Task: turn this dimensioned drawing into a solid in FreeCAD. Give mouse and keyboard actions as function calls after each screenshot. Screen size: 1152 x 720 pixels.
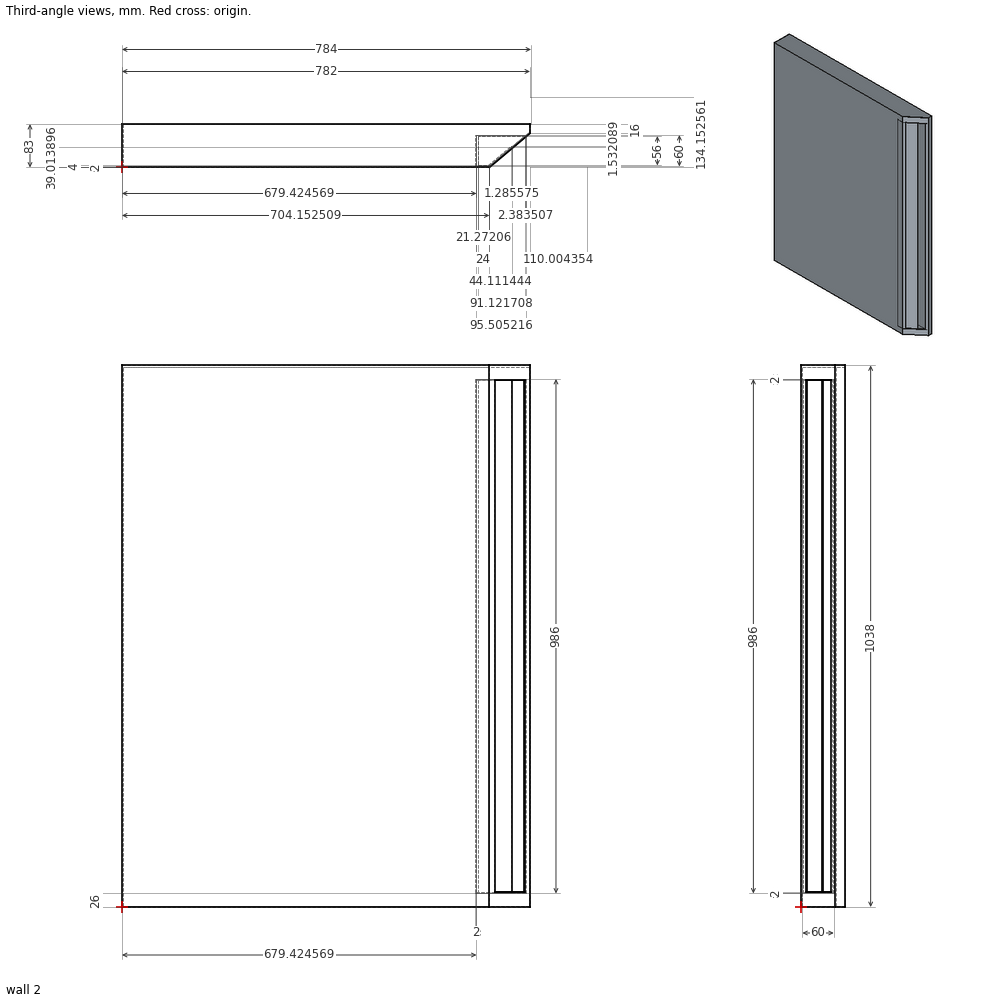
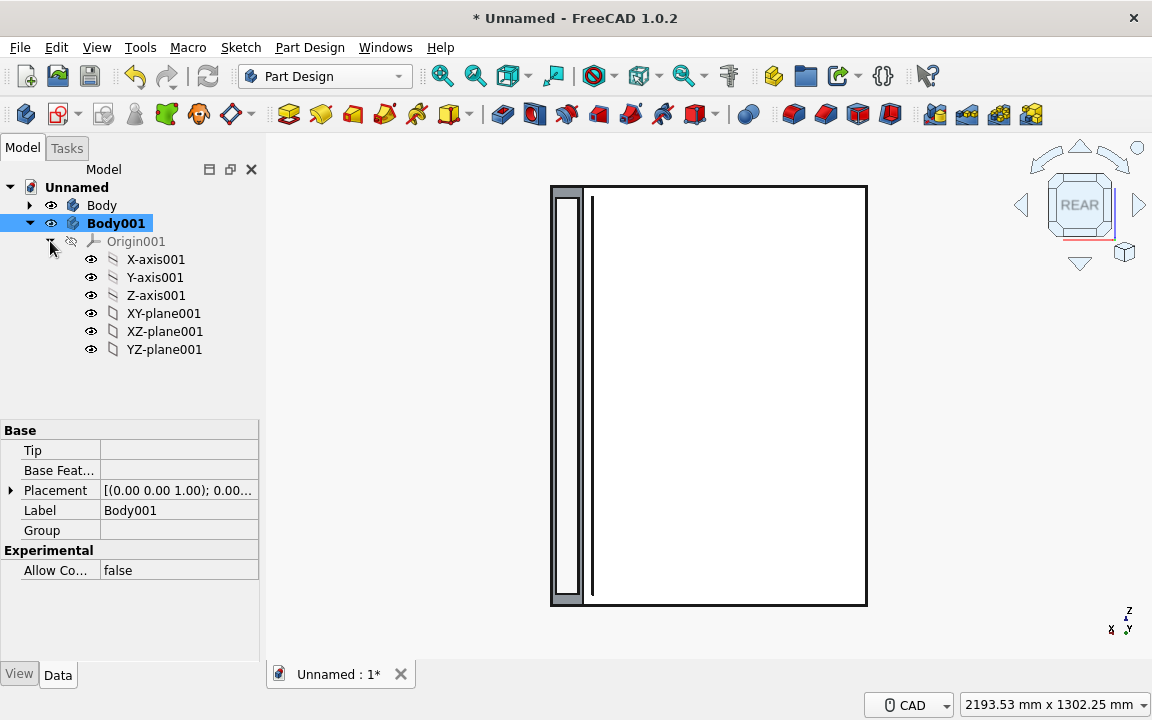
click(136, 313)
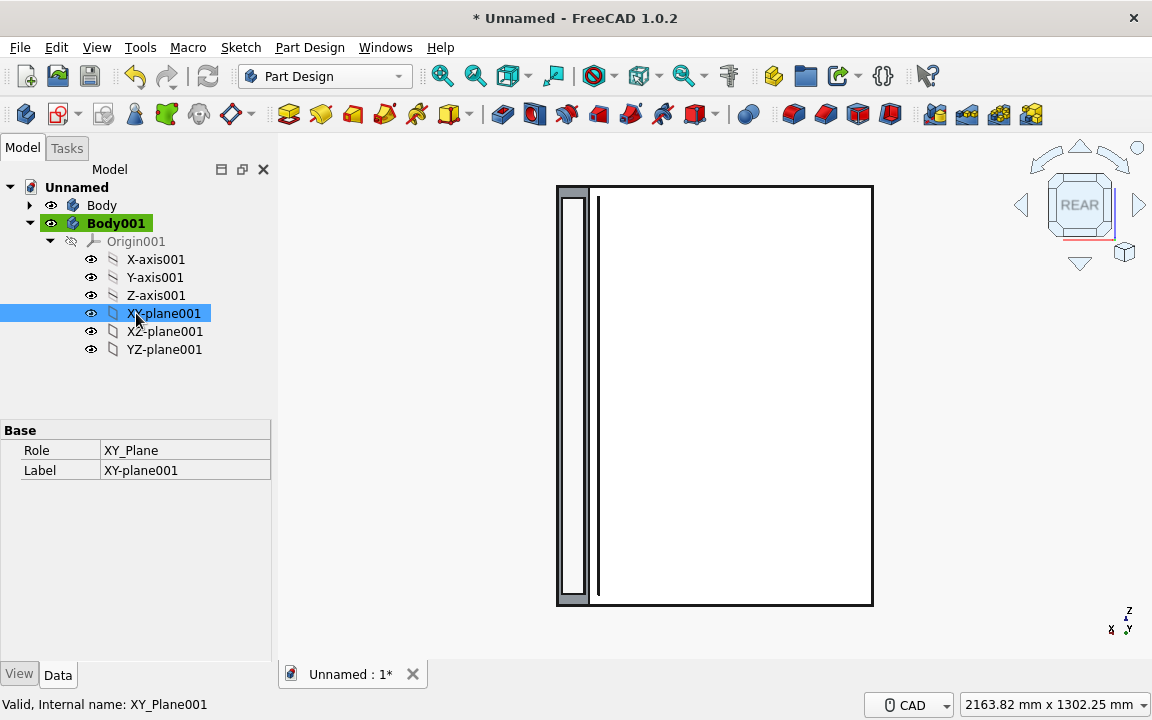
click(232, 114)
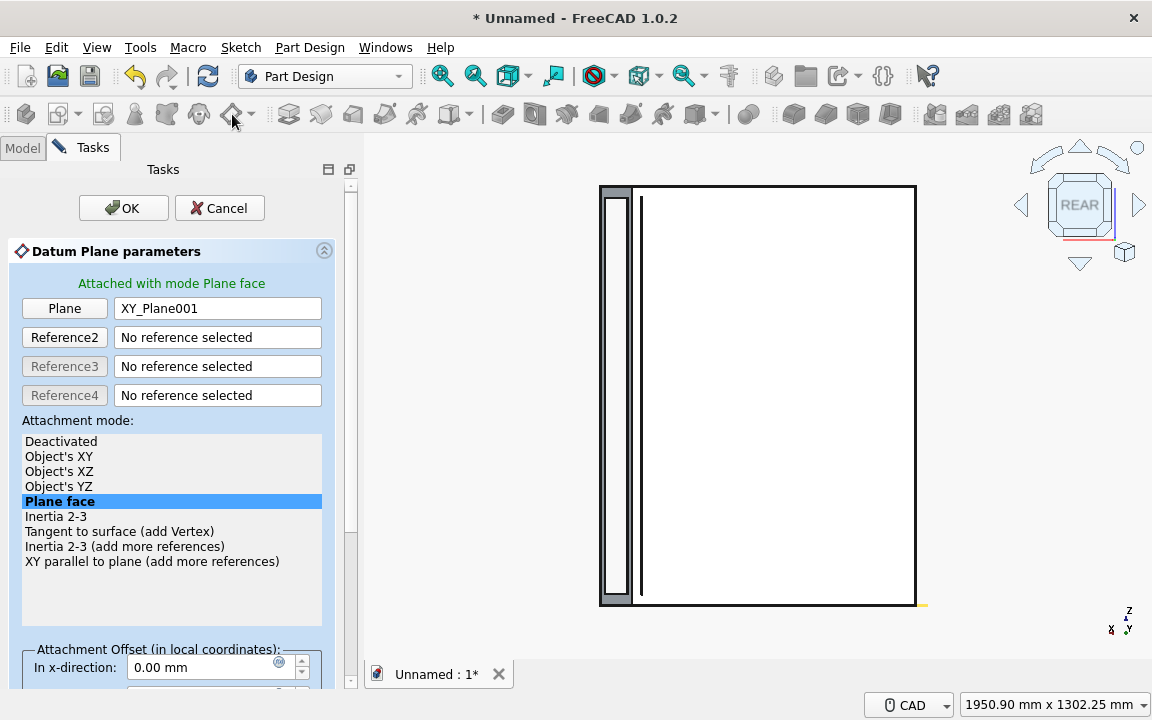
scroll(351, 434, down, 2)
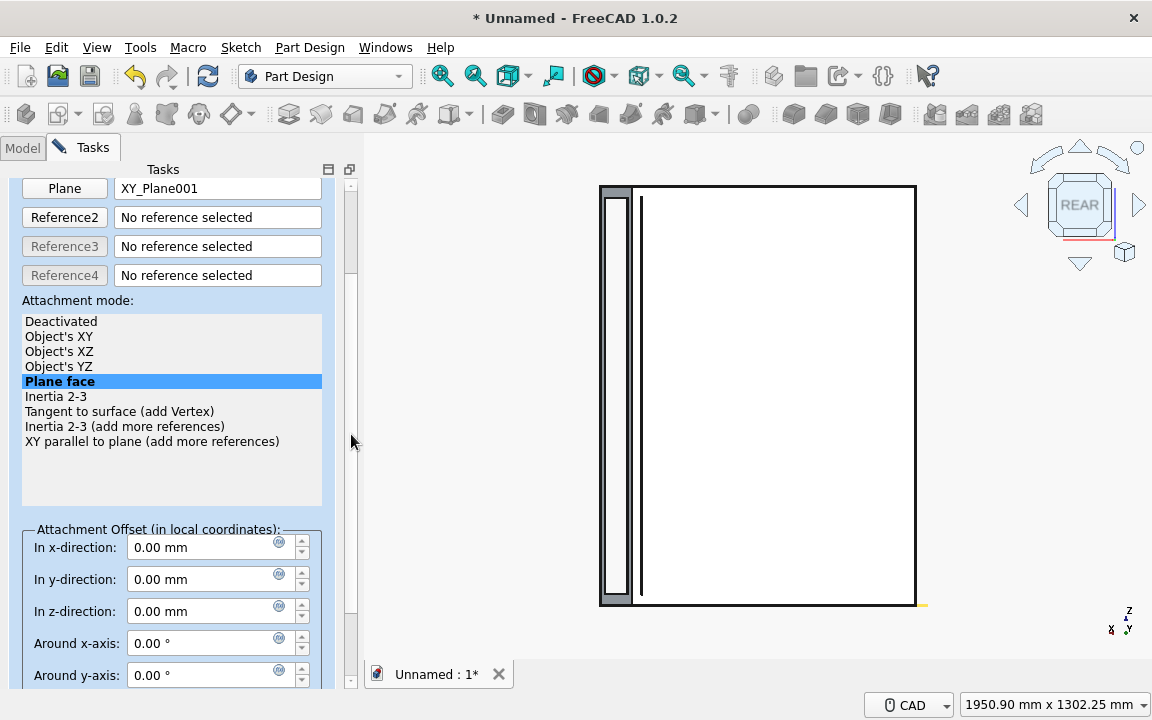
triple_click(210, 611)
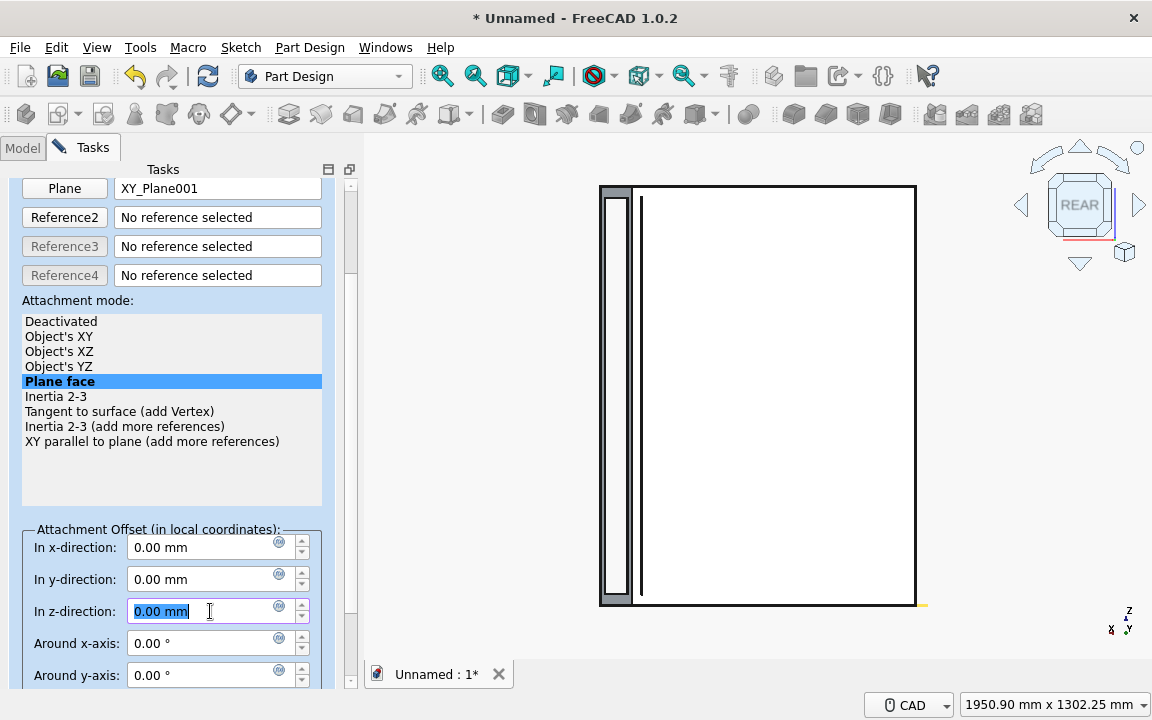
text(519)
key(Tab)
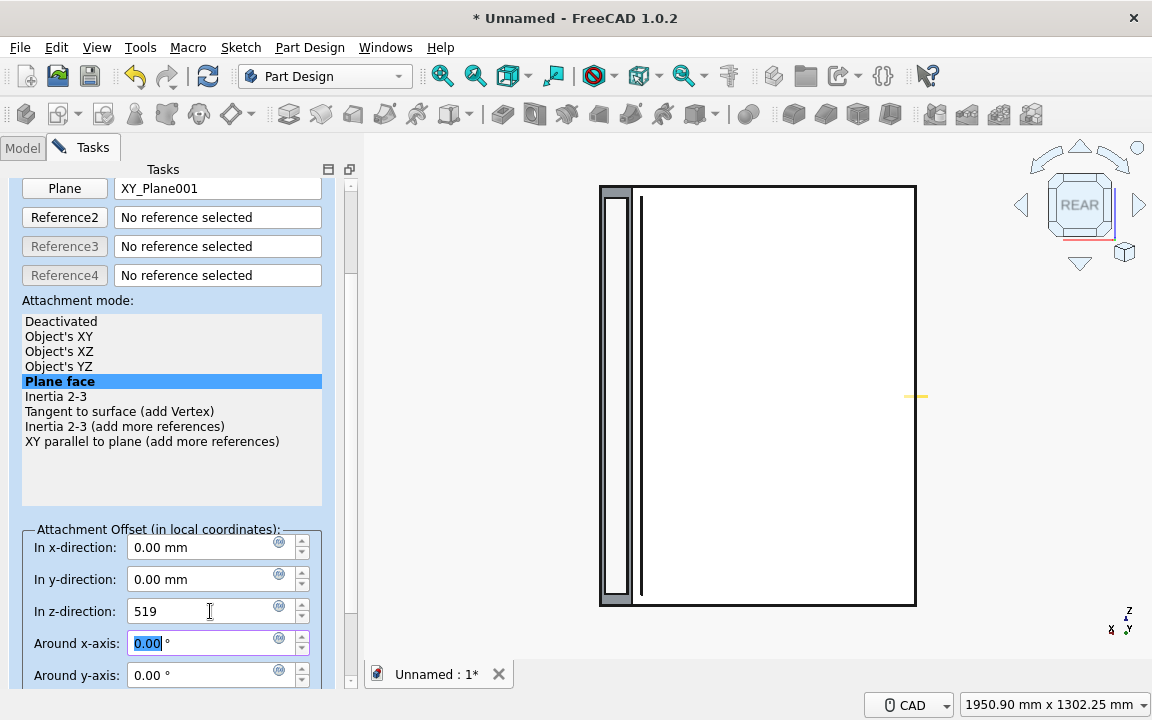
scroll(351, 434, up, 3)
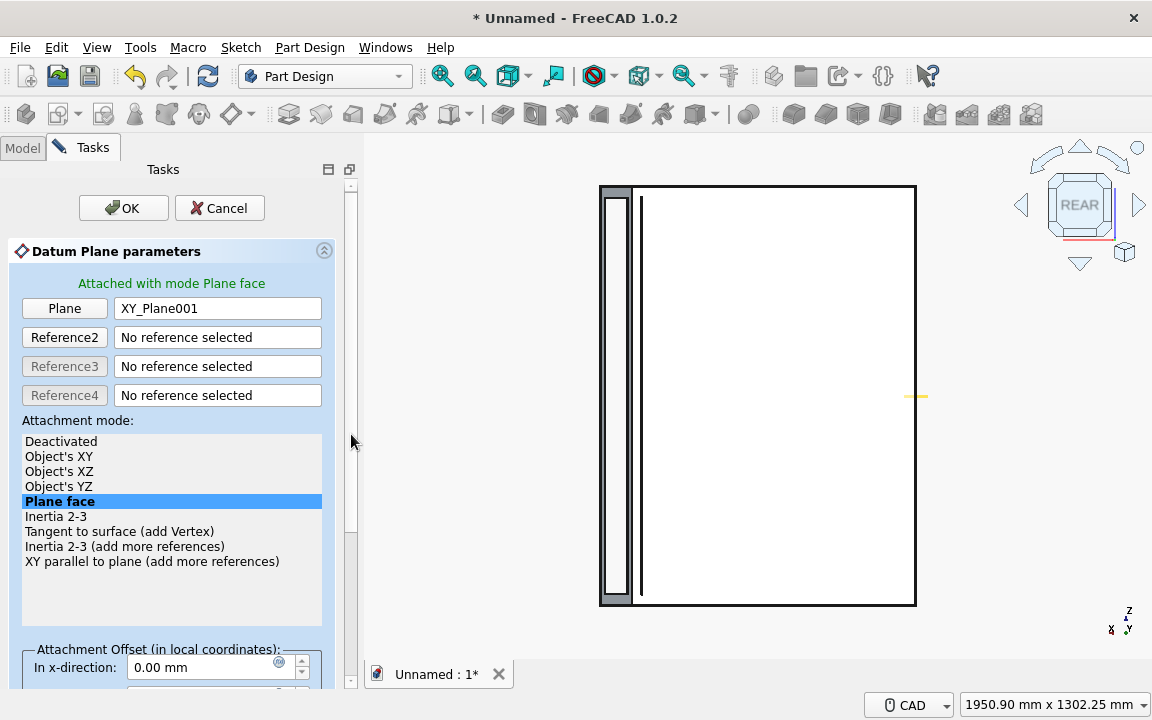
click(124, 208)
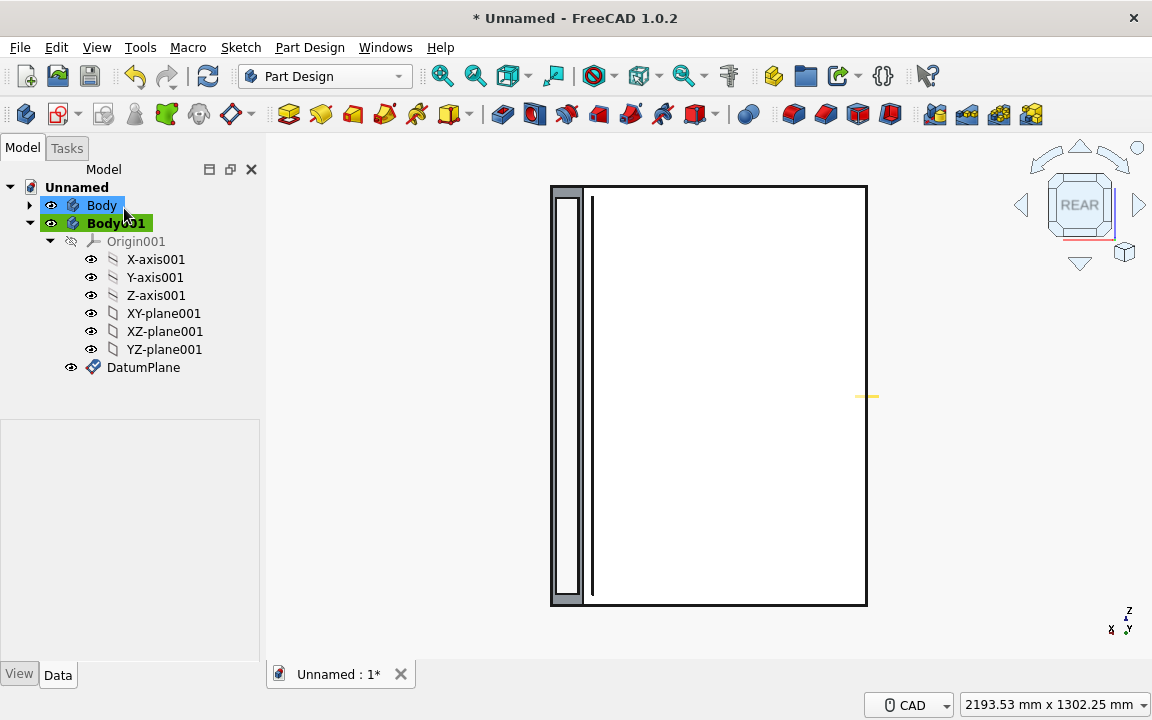
click(116, 367)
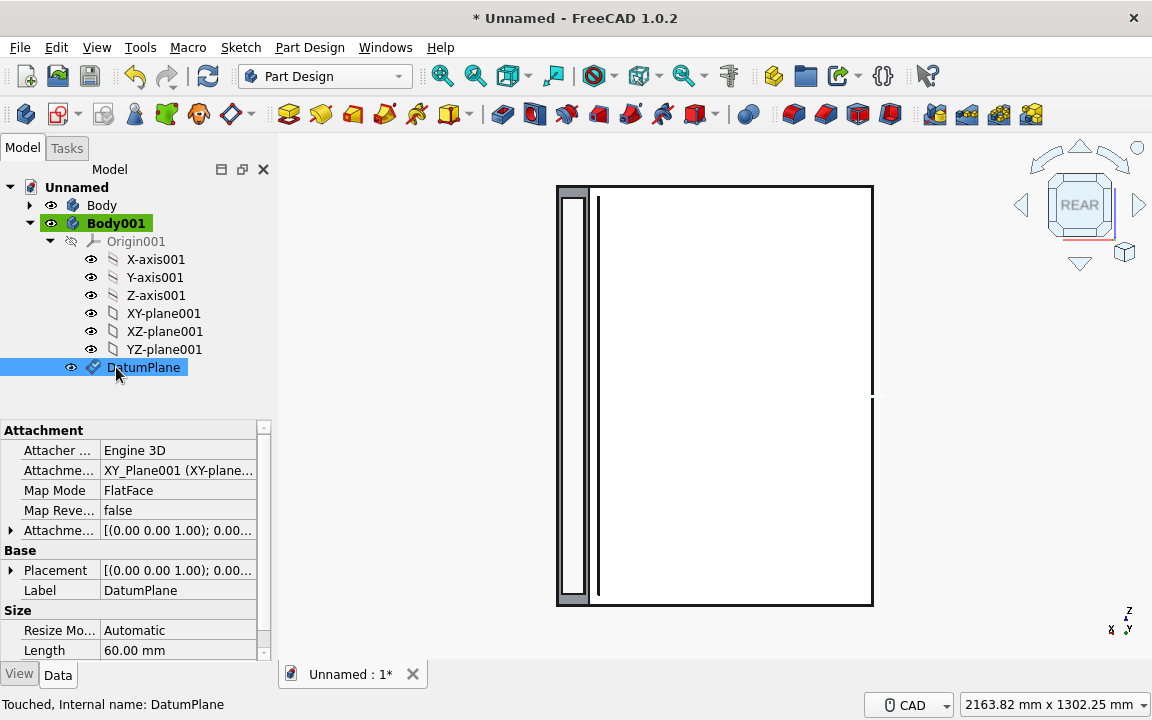
click(58, 114)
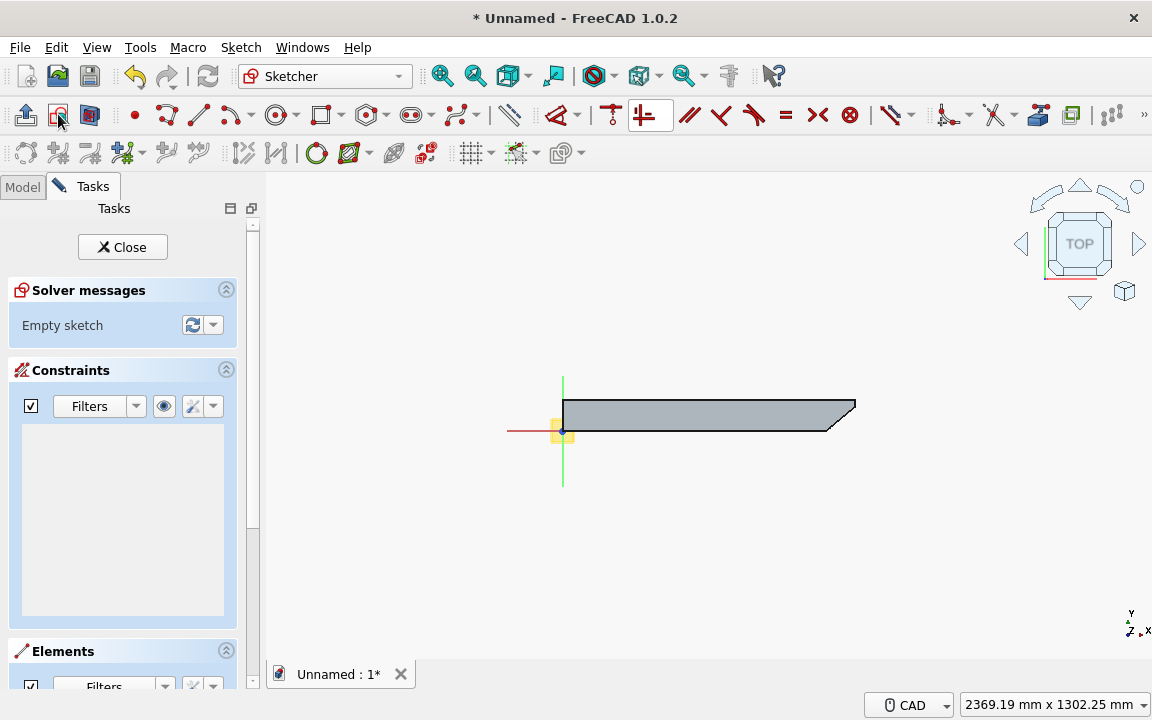
scroll(850, 419, up, 13)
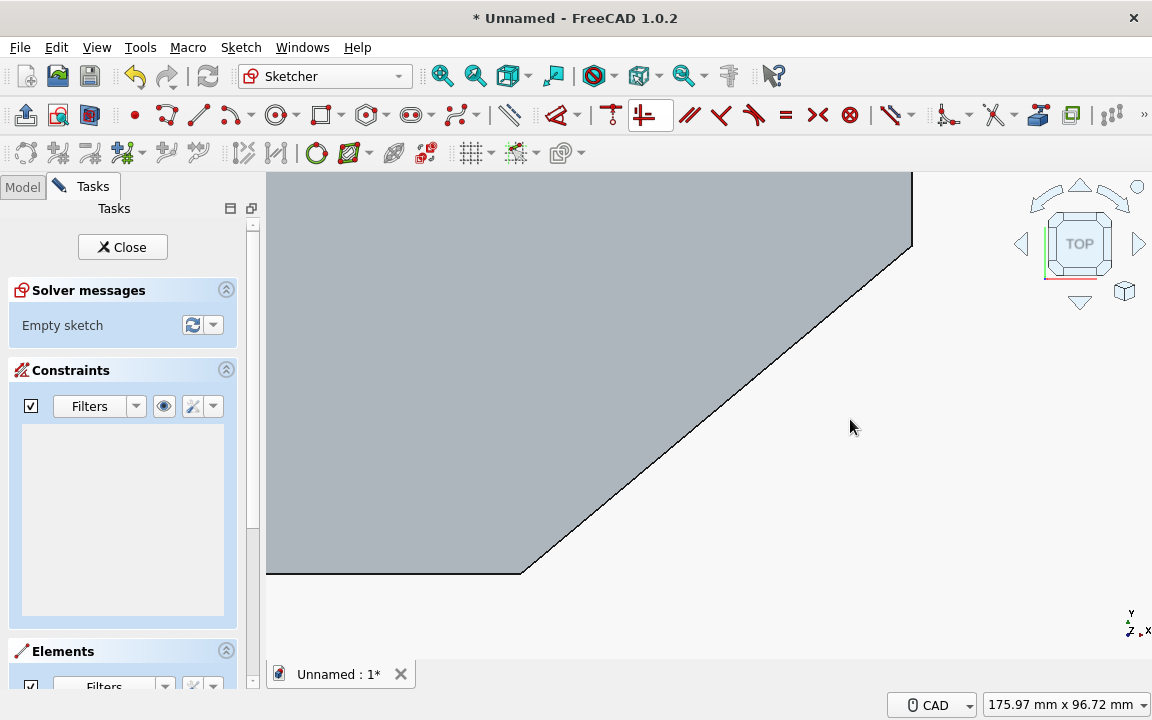
key(g)
key(m)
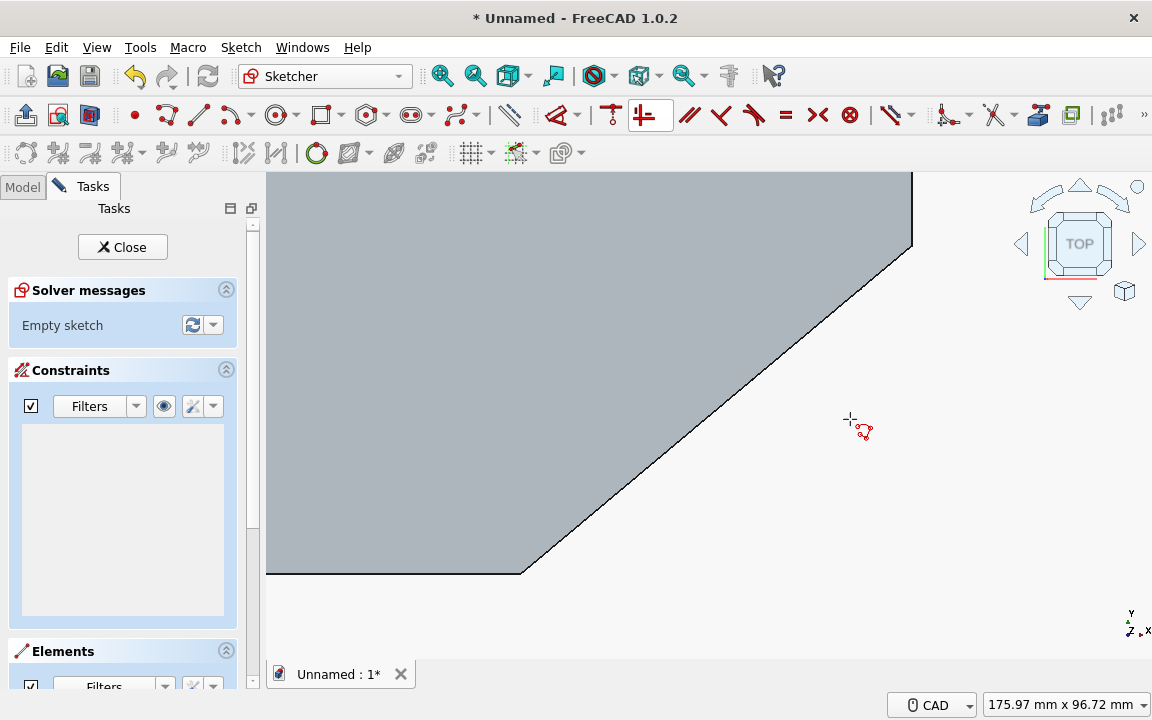
scroll(396, 564, up, 3)